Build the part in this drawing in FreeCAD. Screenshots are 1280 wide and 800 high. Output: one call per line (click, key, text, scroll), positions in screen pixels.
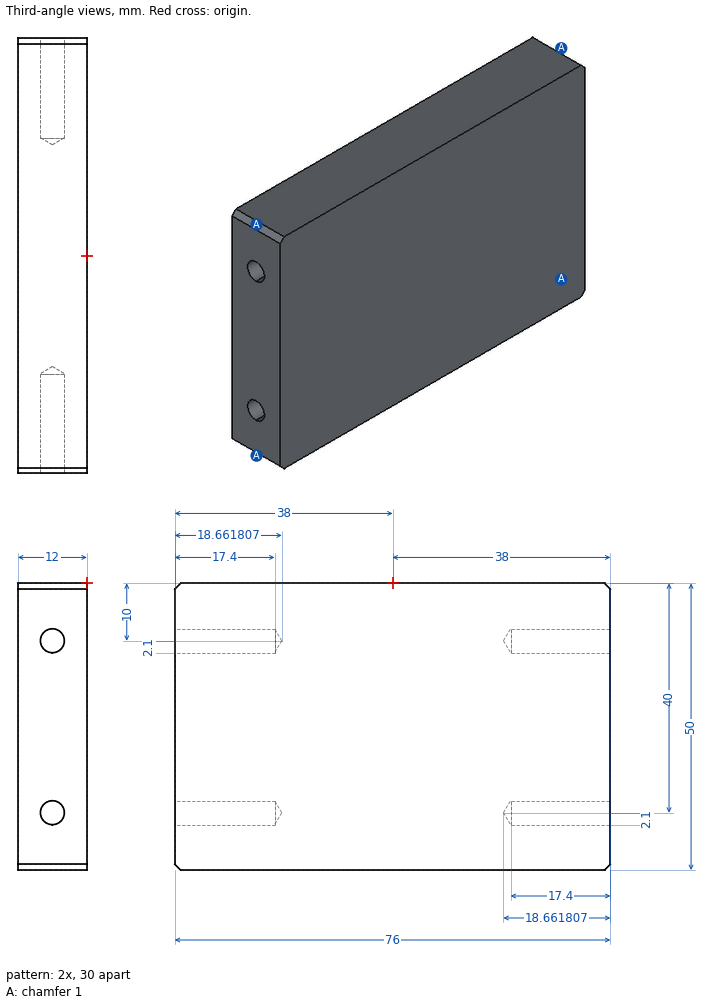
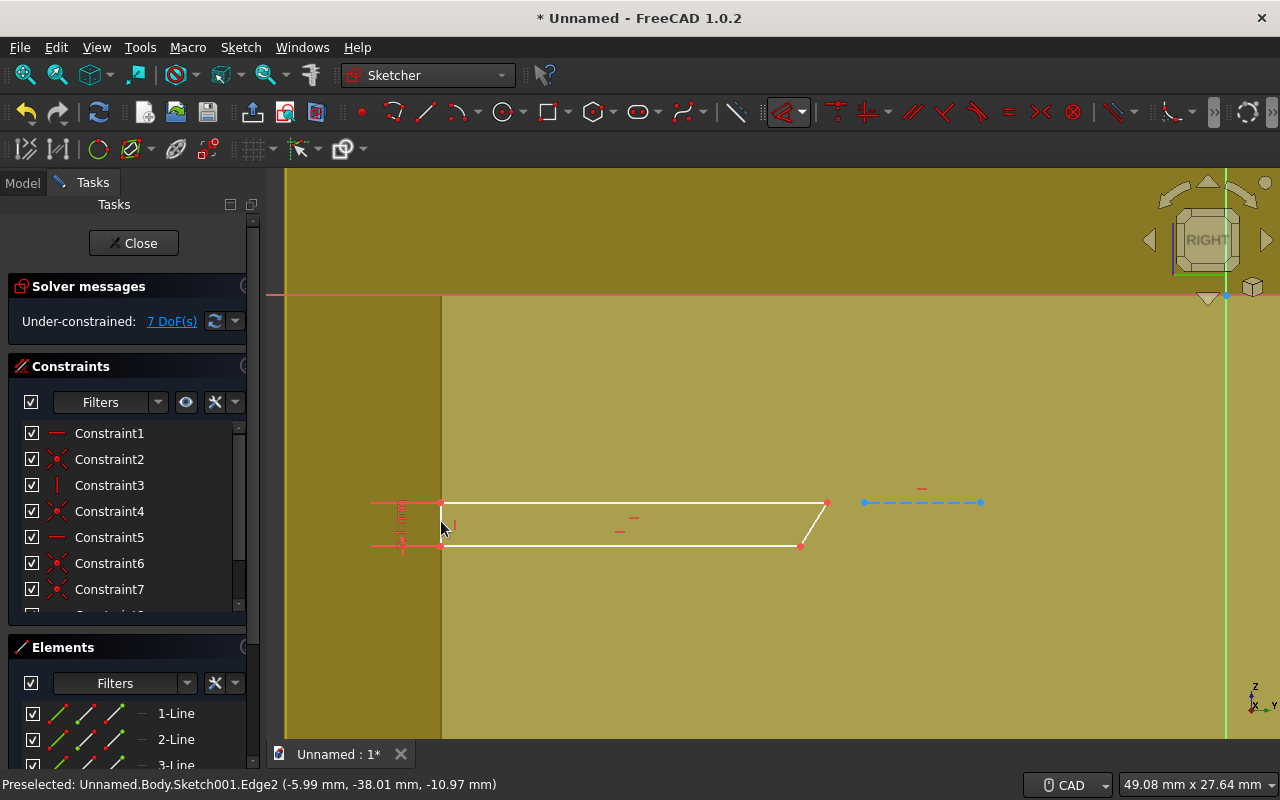
click(827, 503)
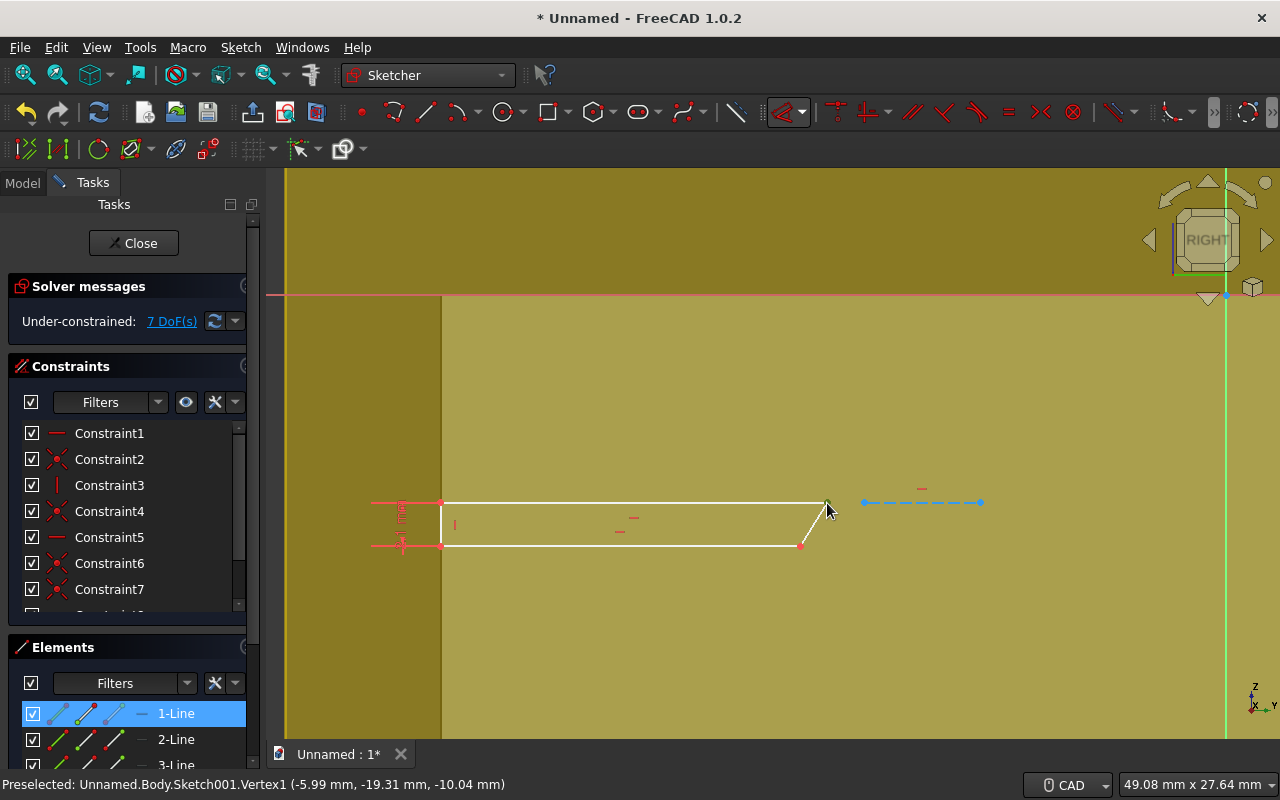
click(804, 112)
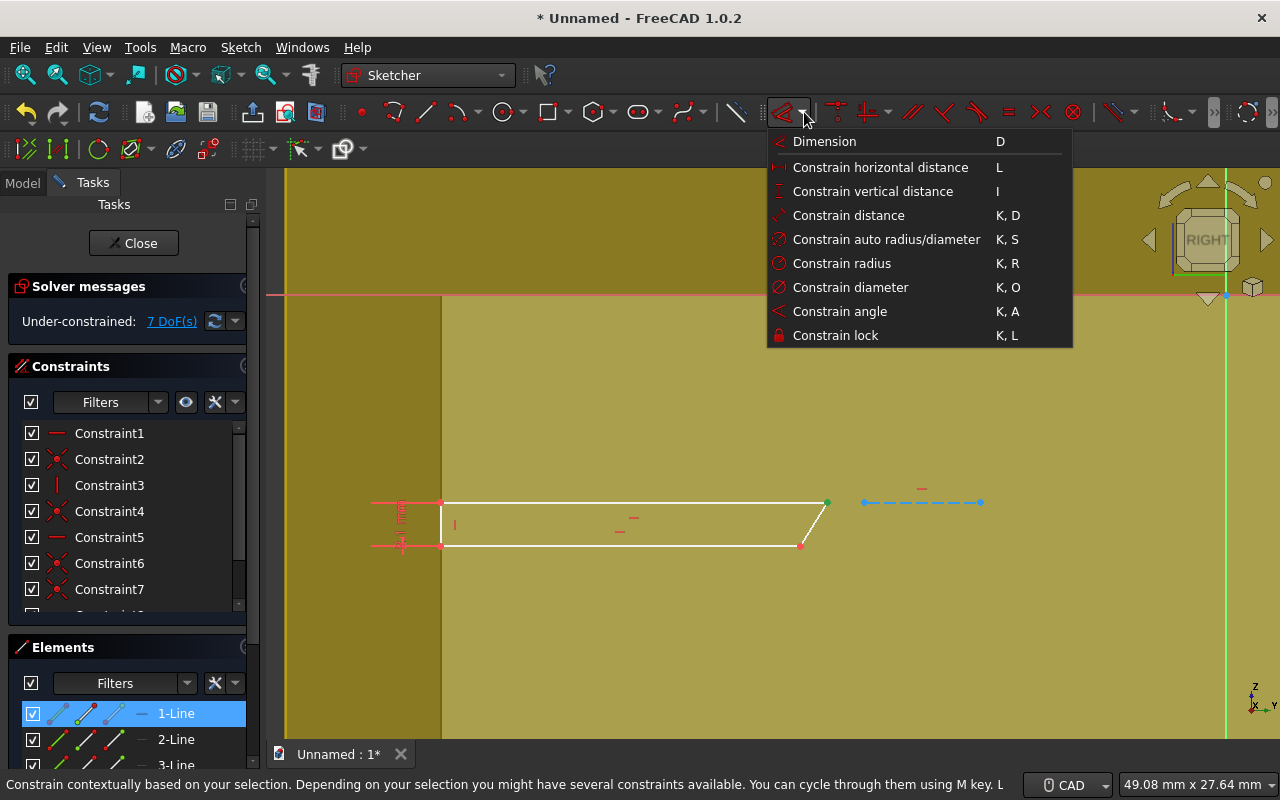
click(920, 191)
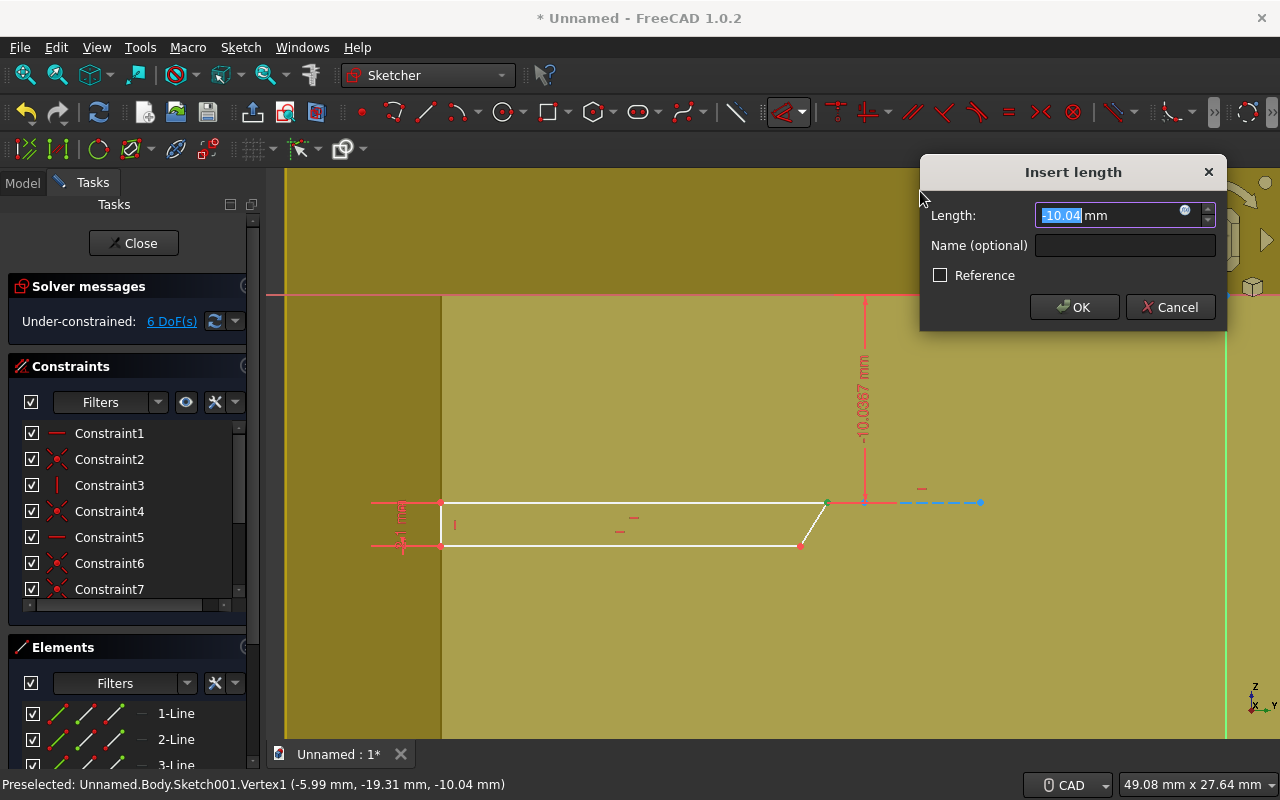
text(-10)
key(Return)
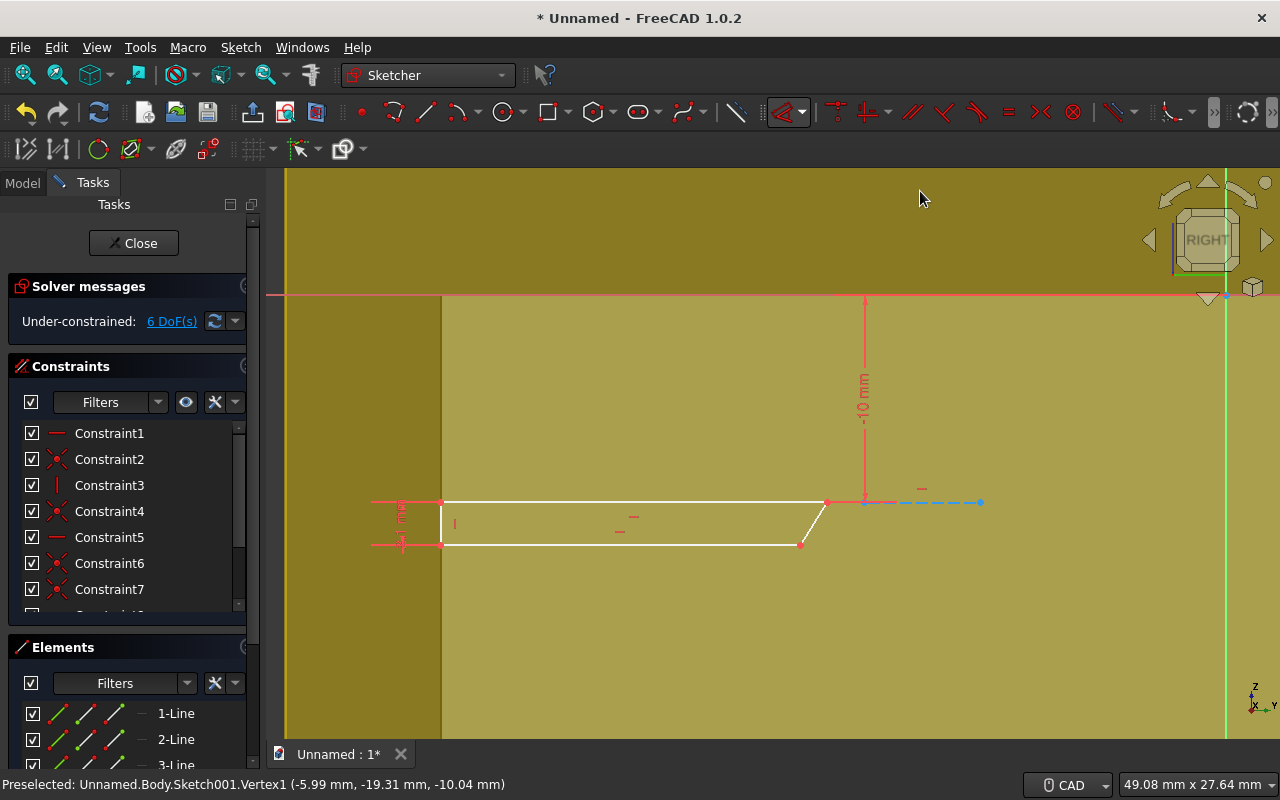
click(441, 502)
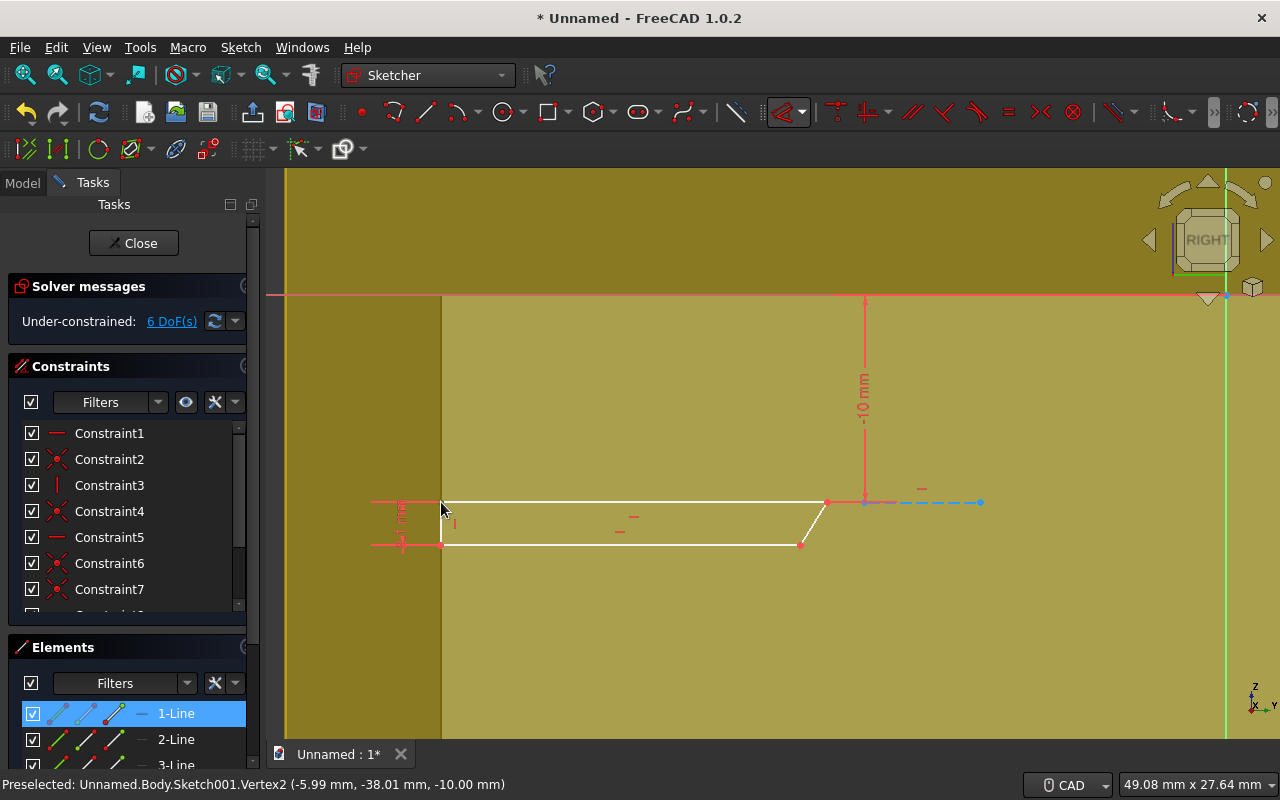
key(l)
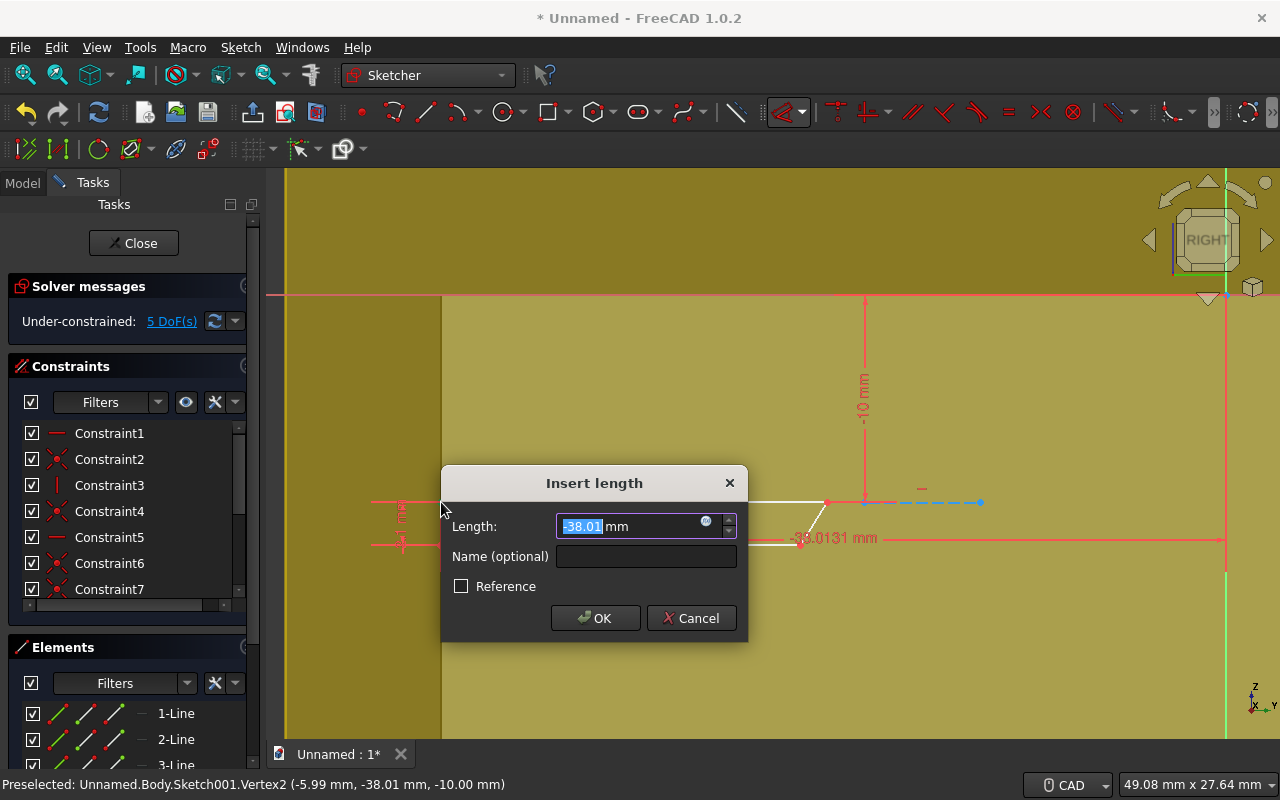
text(-38)
key(Return)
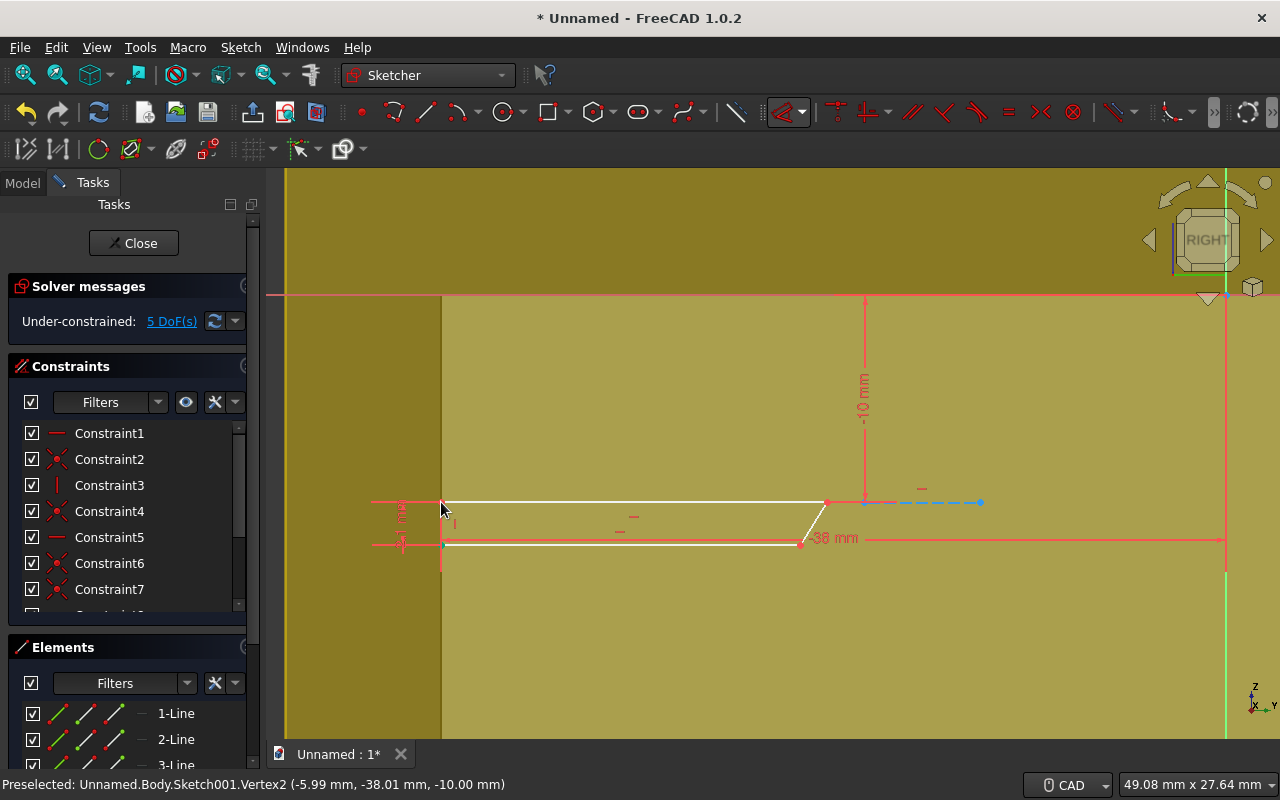
click(865, 503)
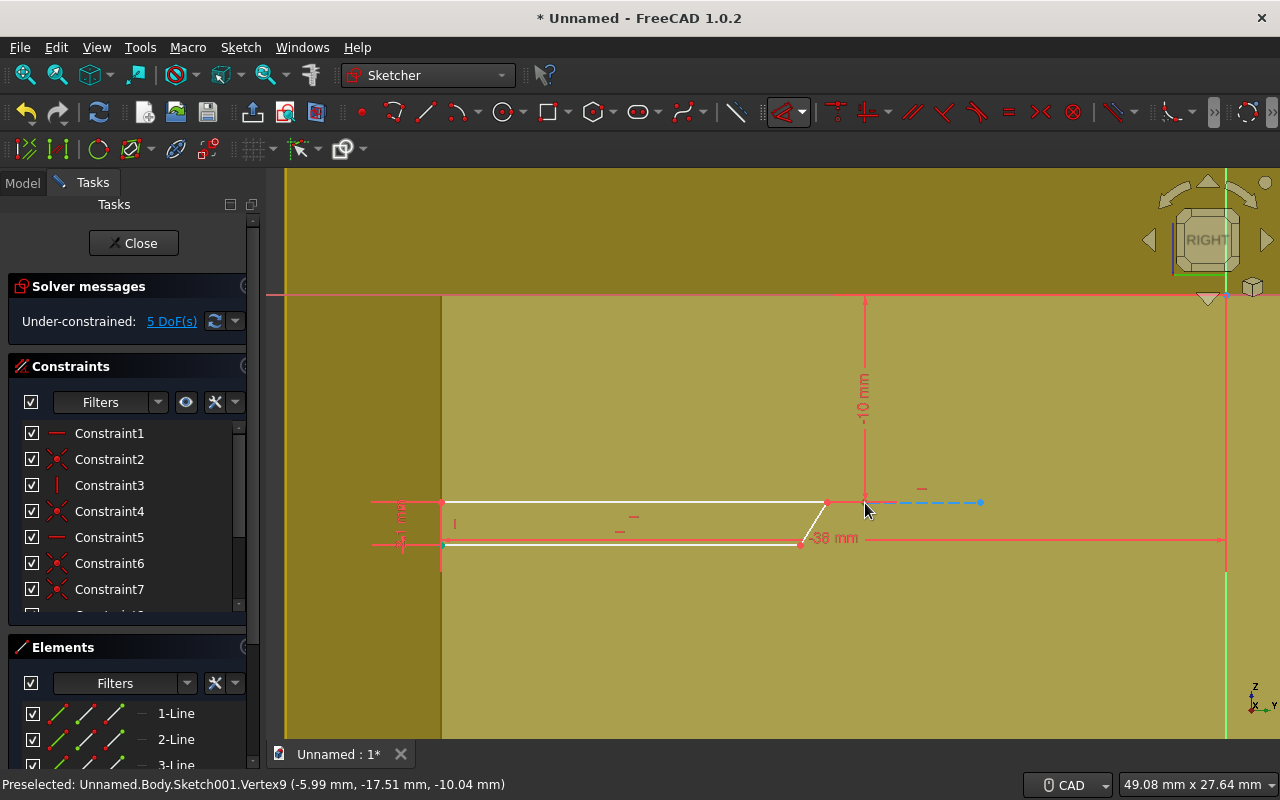
click(804, 112)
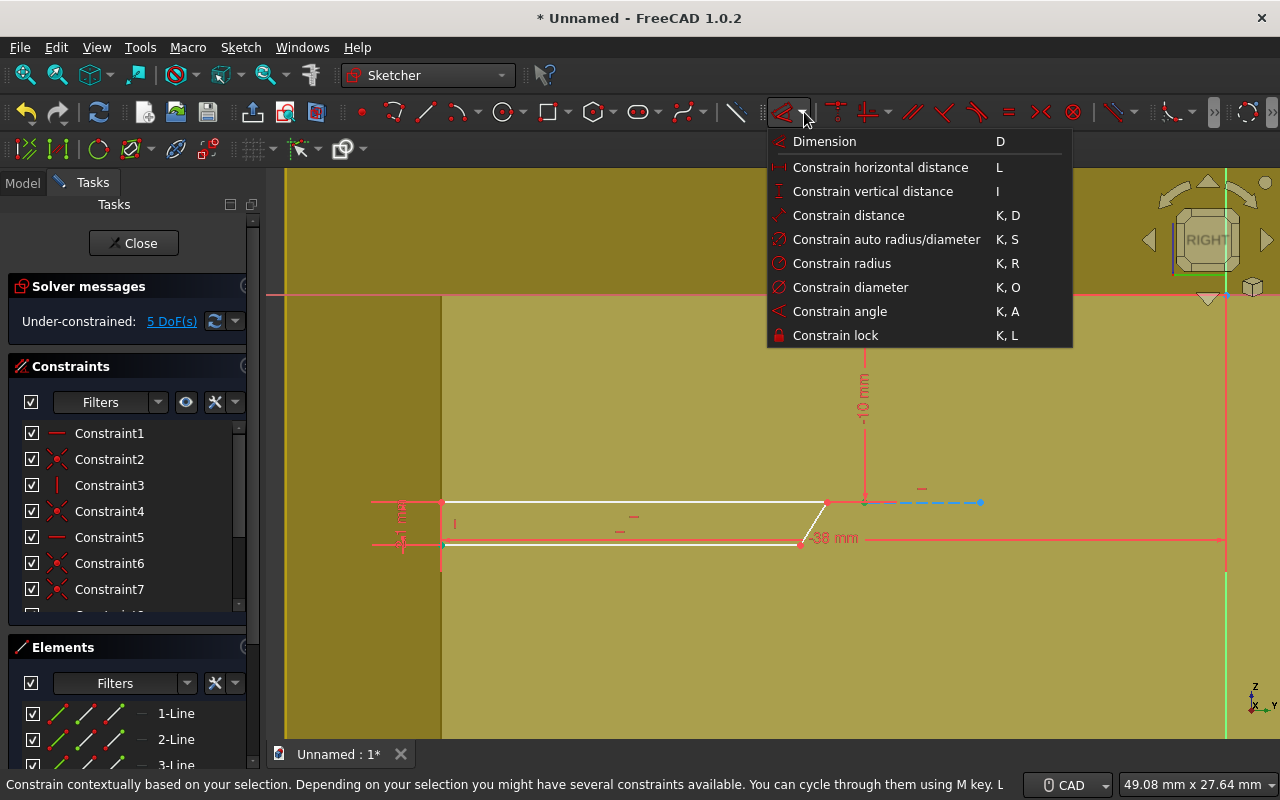
click(920, 191)